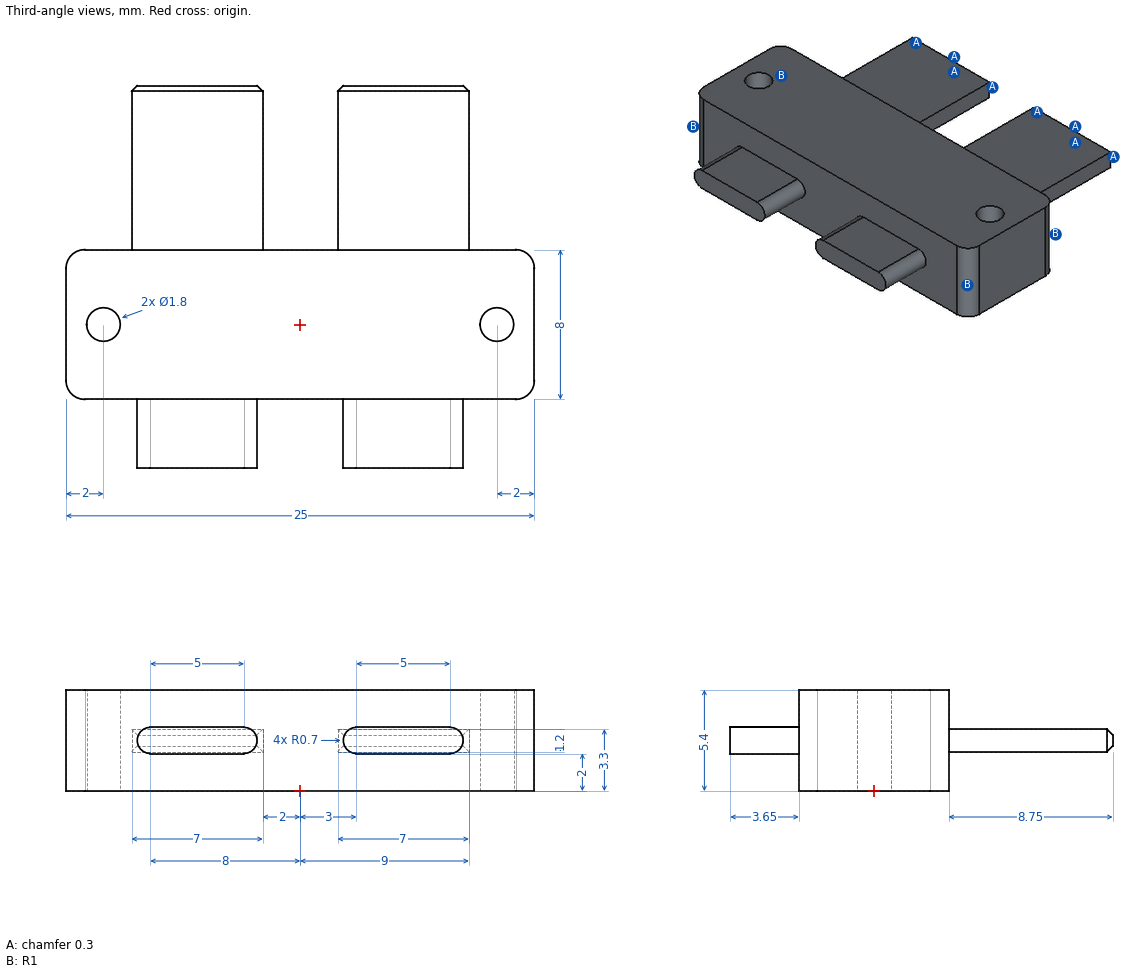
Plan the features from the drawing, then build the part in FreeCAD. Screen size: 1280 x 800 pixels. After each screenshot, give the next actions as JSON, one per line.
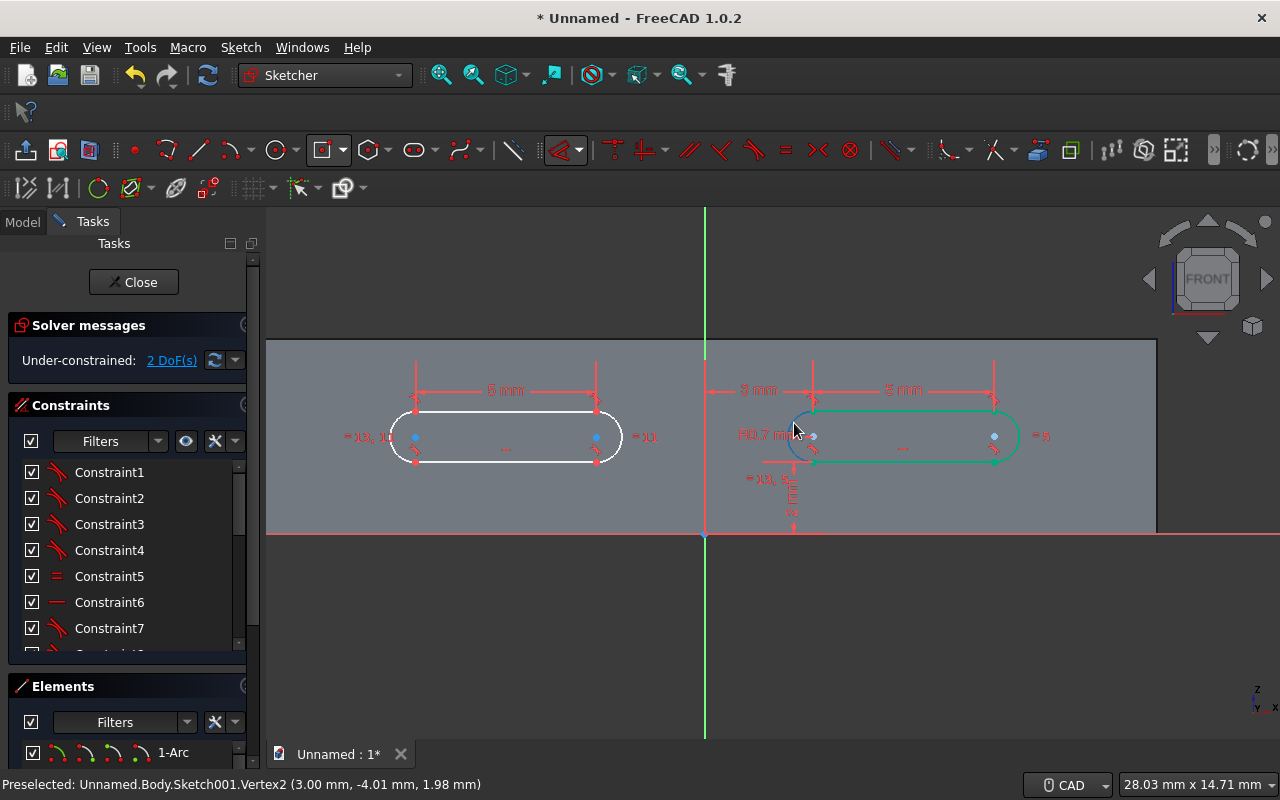
{"action": "left_click", "coordinate": [416, 412]}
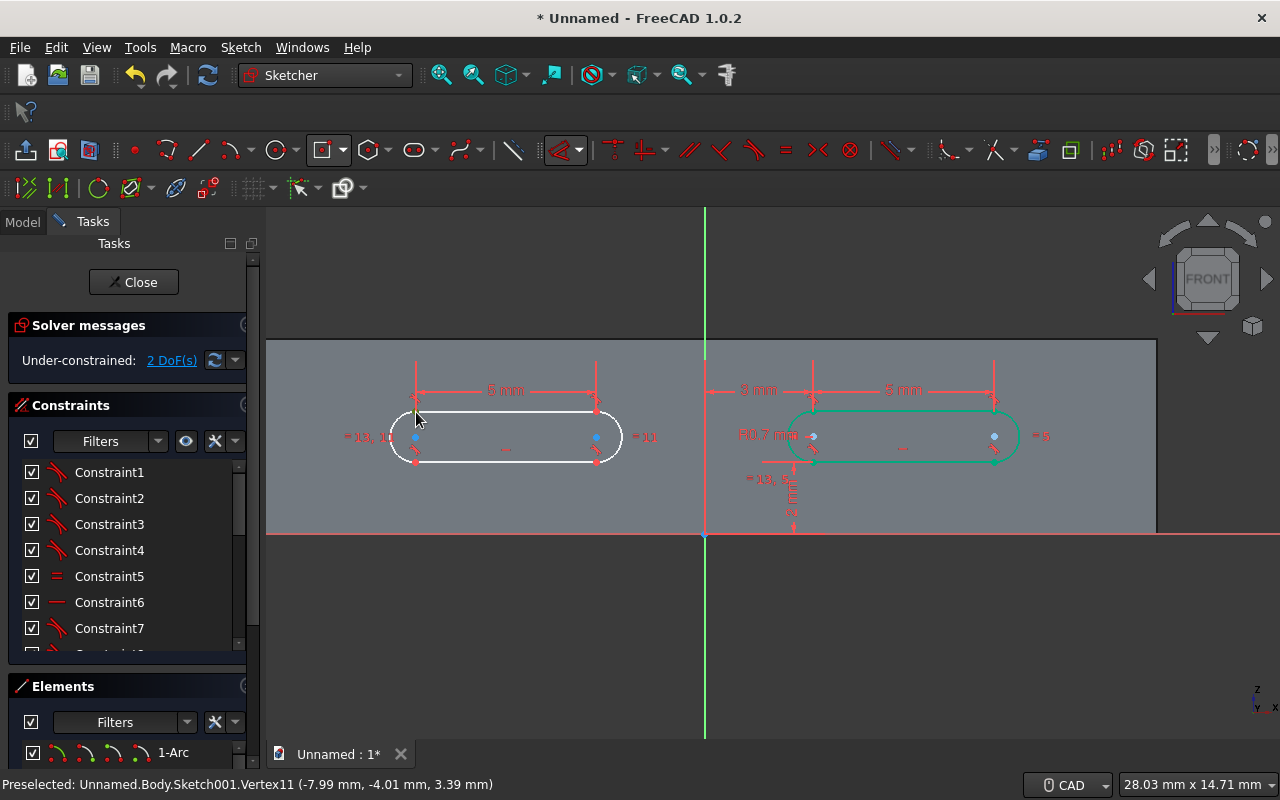
{"action": "left_click", "coordinate": [582, 150]}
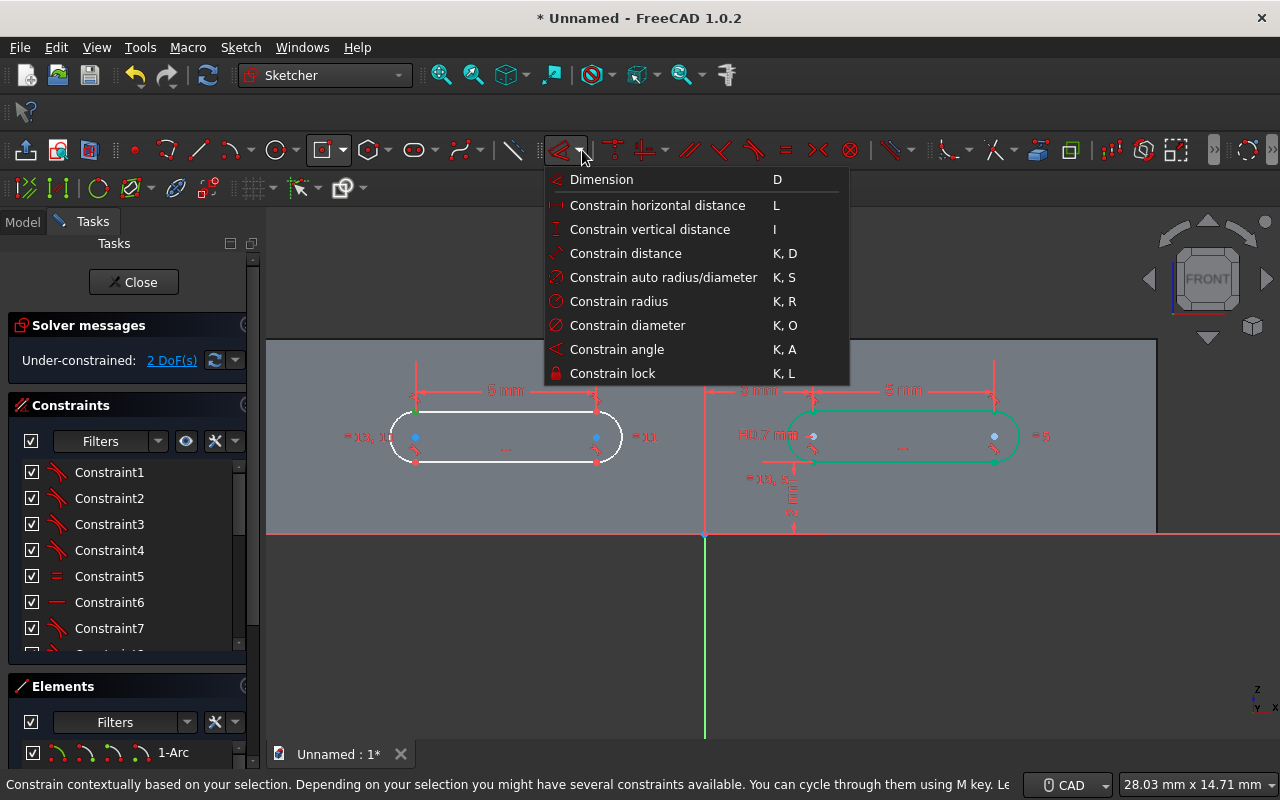
{"action": "left_click", "coordinate": [697, 205]}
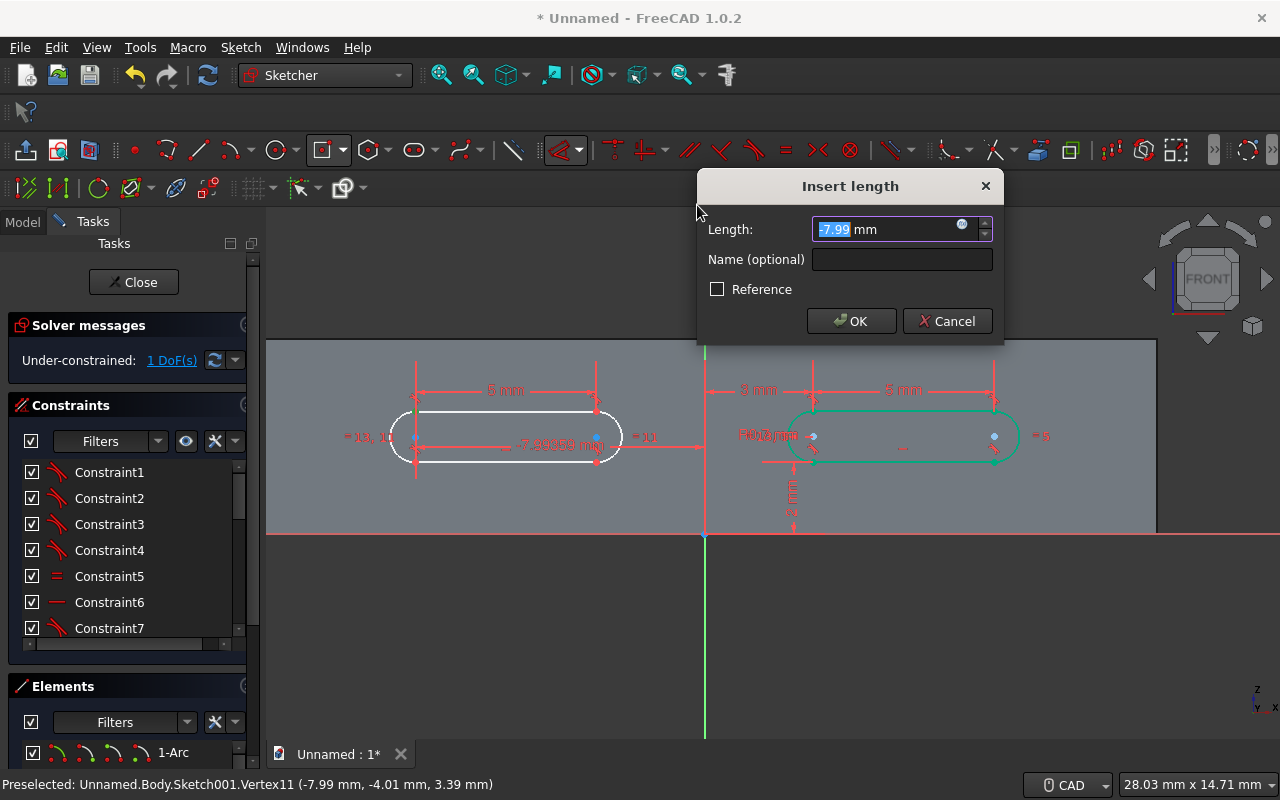
{"action": "type", "text": "-8"}
{"action": "key", "text": "Return"}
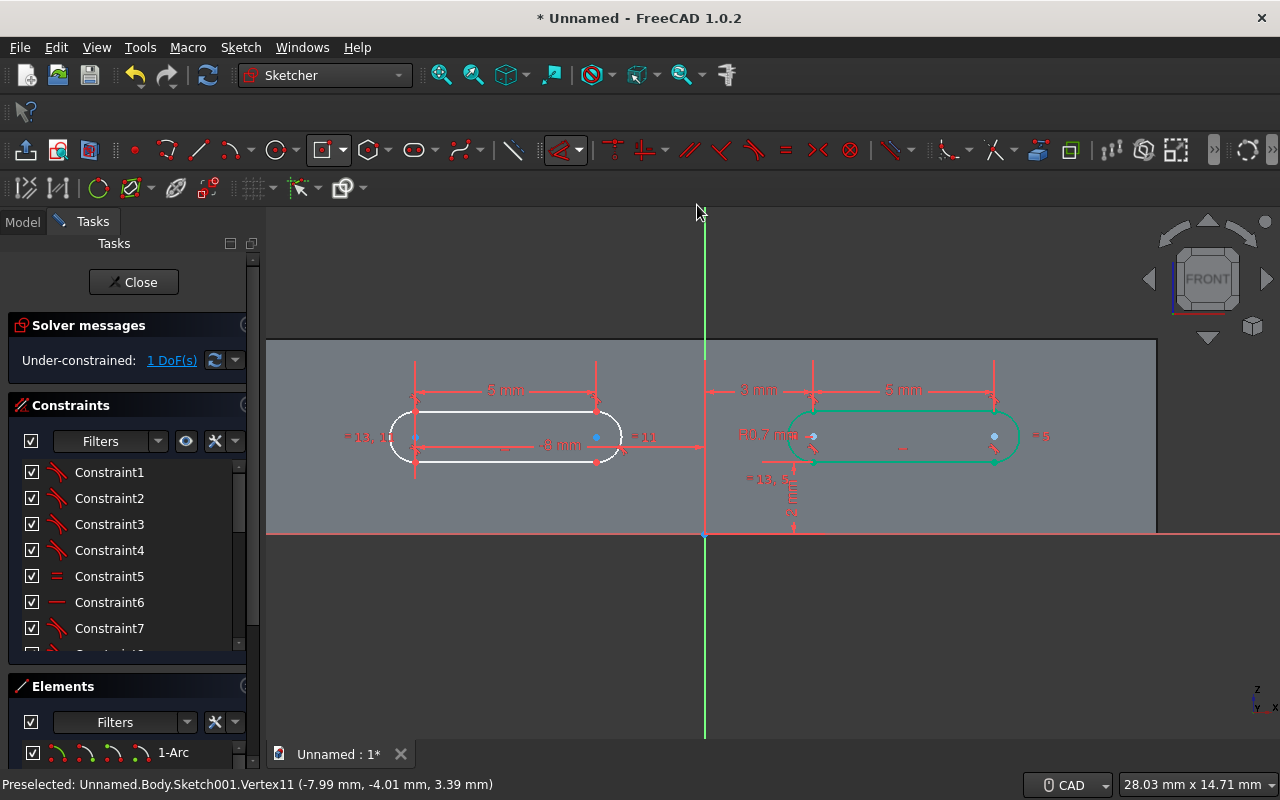
{"action": "left_click", "coordinate": [415, 462]}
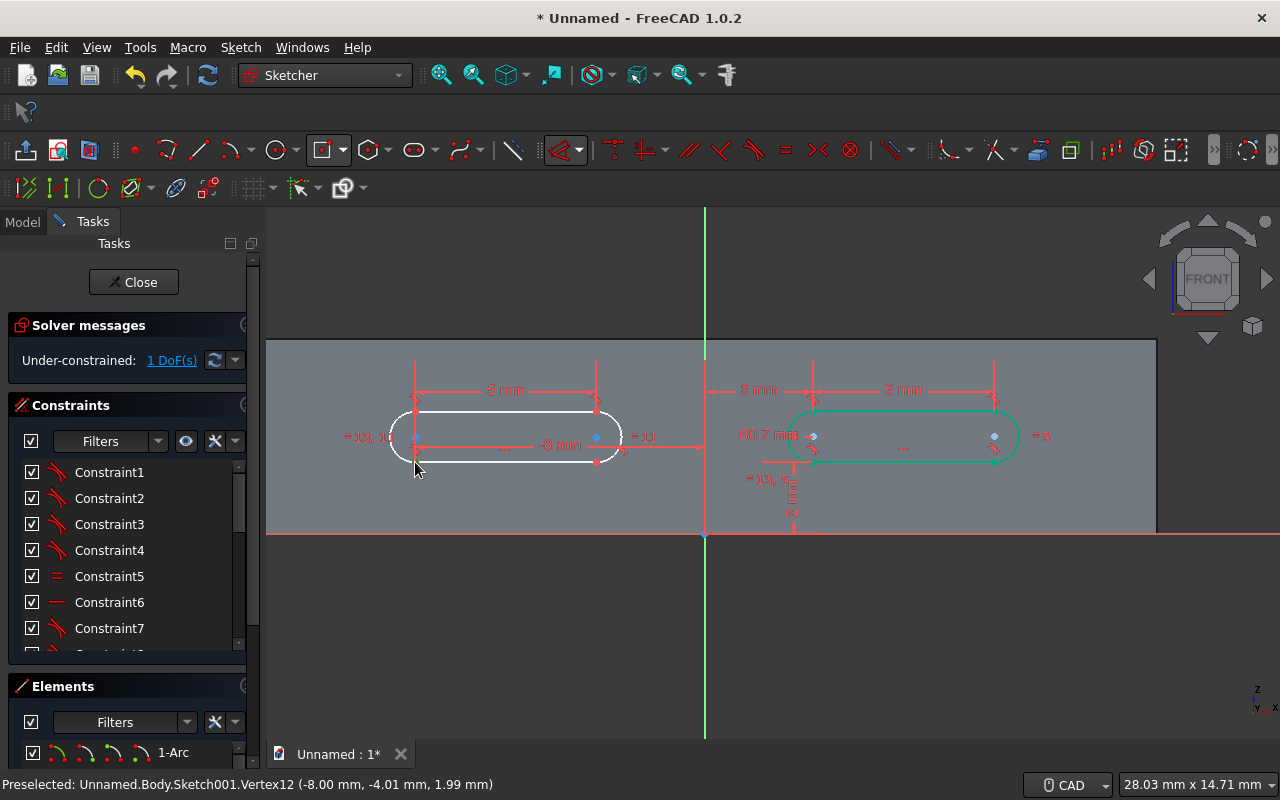
{"action": "key", "text": "i"}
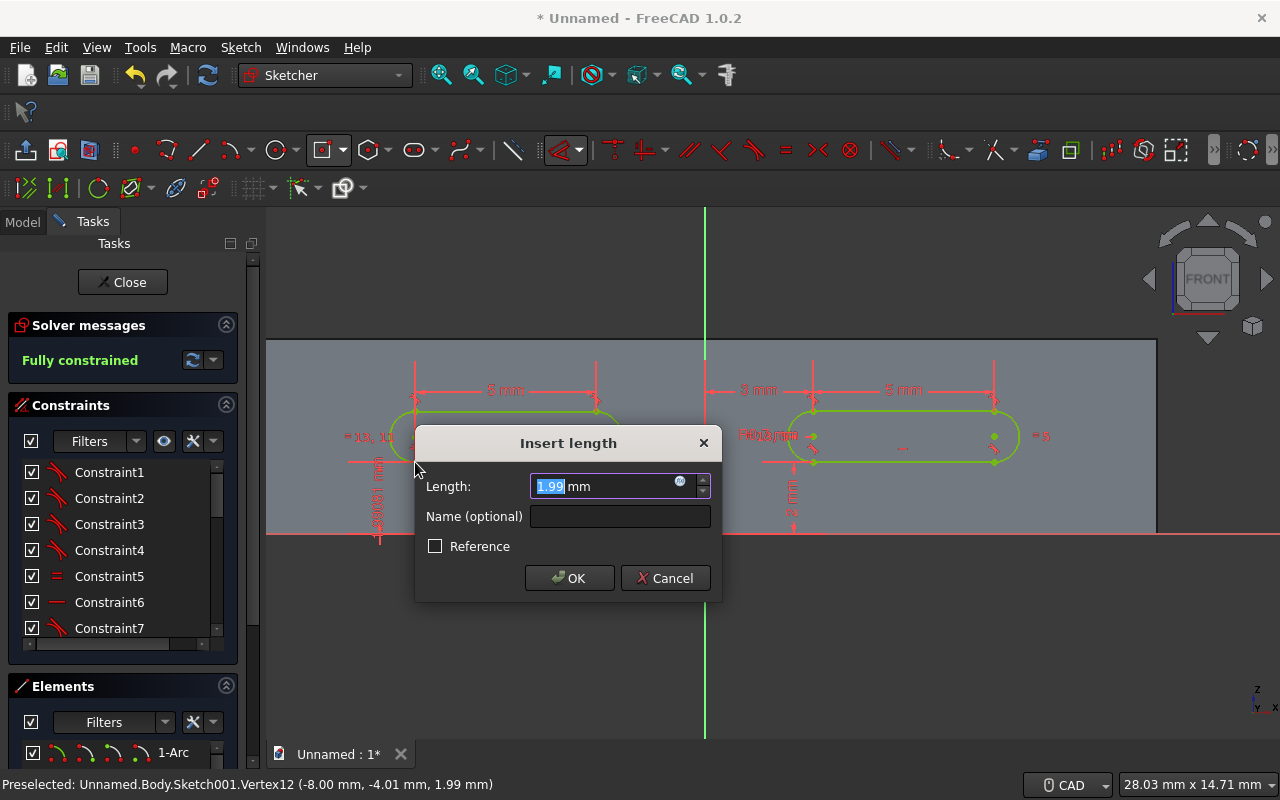
{"action": "type", "text": "2"}
{"action": "key", "text": "Return"}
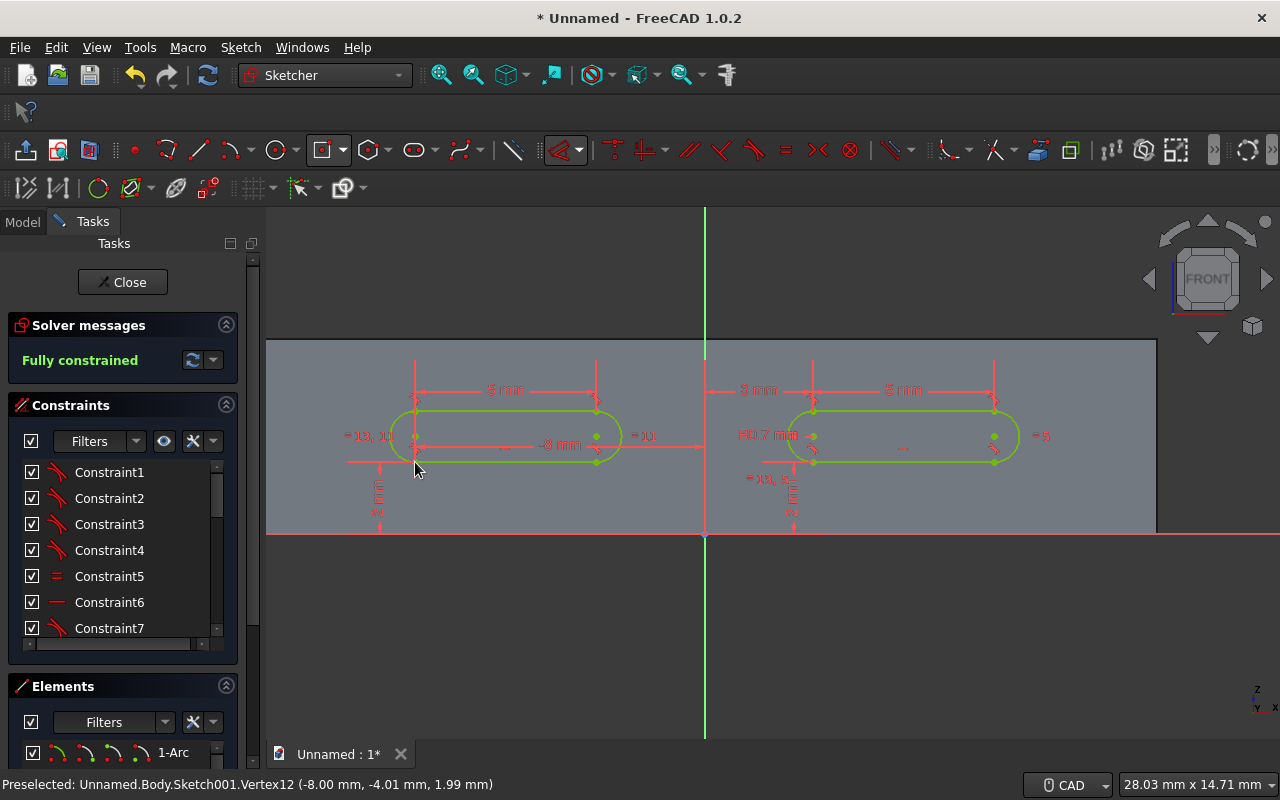
{"action": "left_click", "coordinate": [123, 282]}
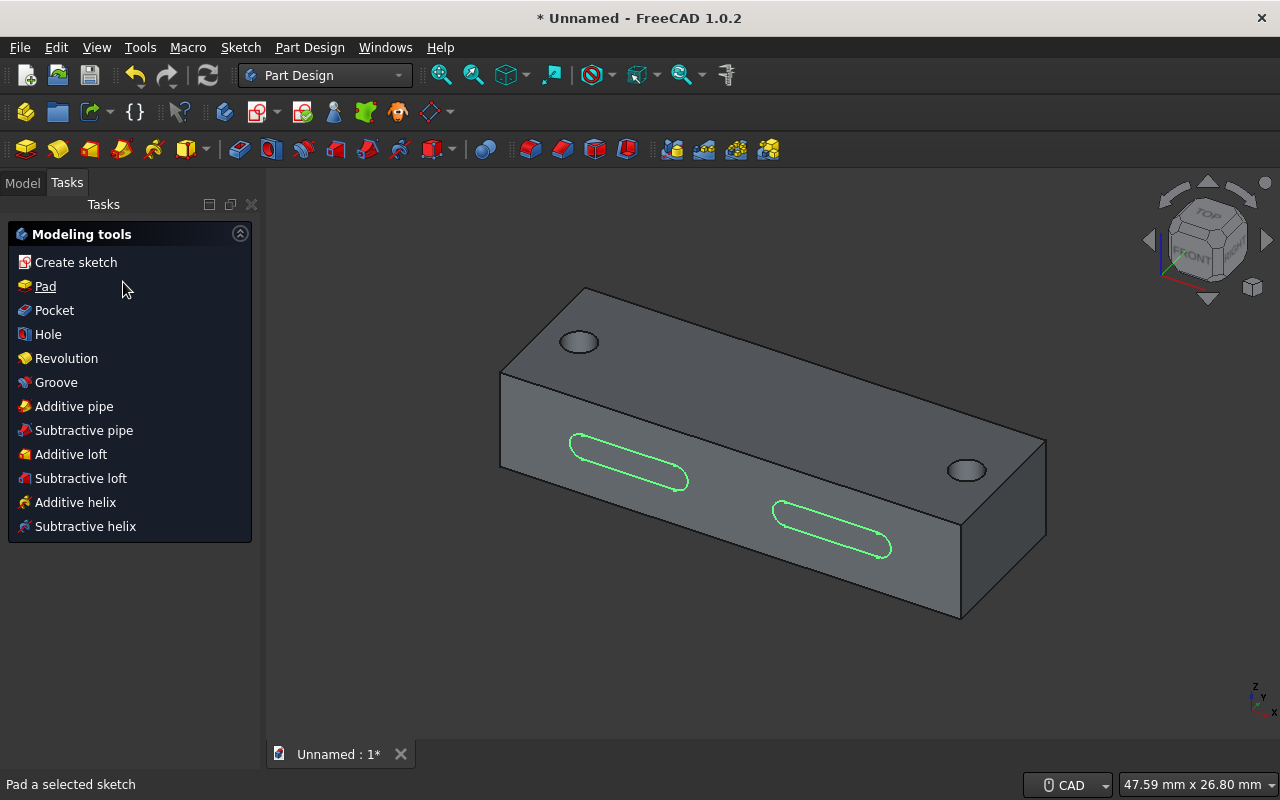
{"action": "left_click", "coordinate": [26, 150]}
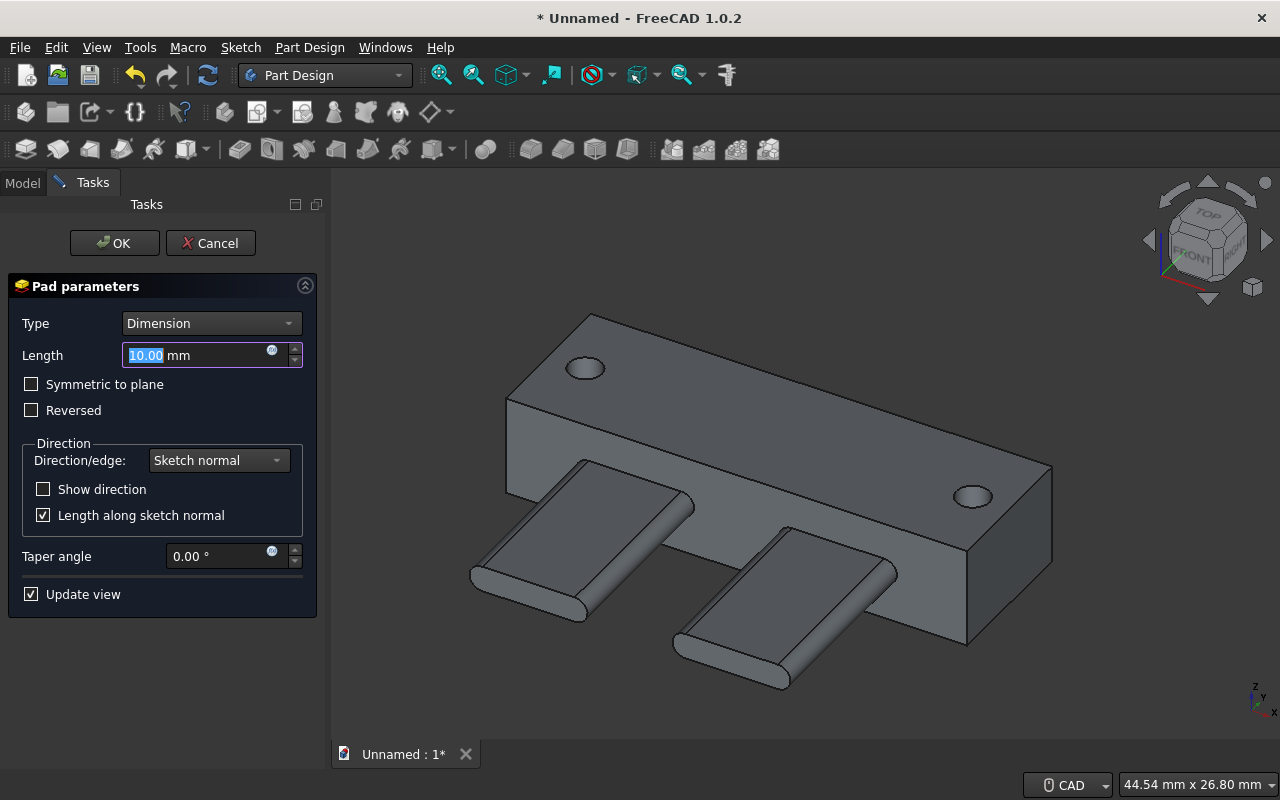
{"action": "type", "text": "3.65"}
{"action": "key", "text": "Tab"}